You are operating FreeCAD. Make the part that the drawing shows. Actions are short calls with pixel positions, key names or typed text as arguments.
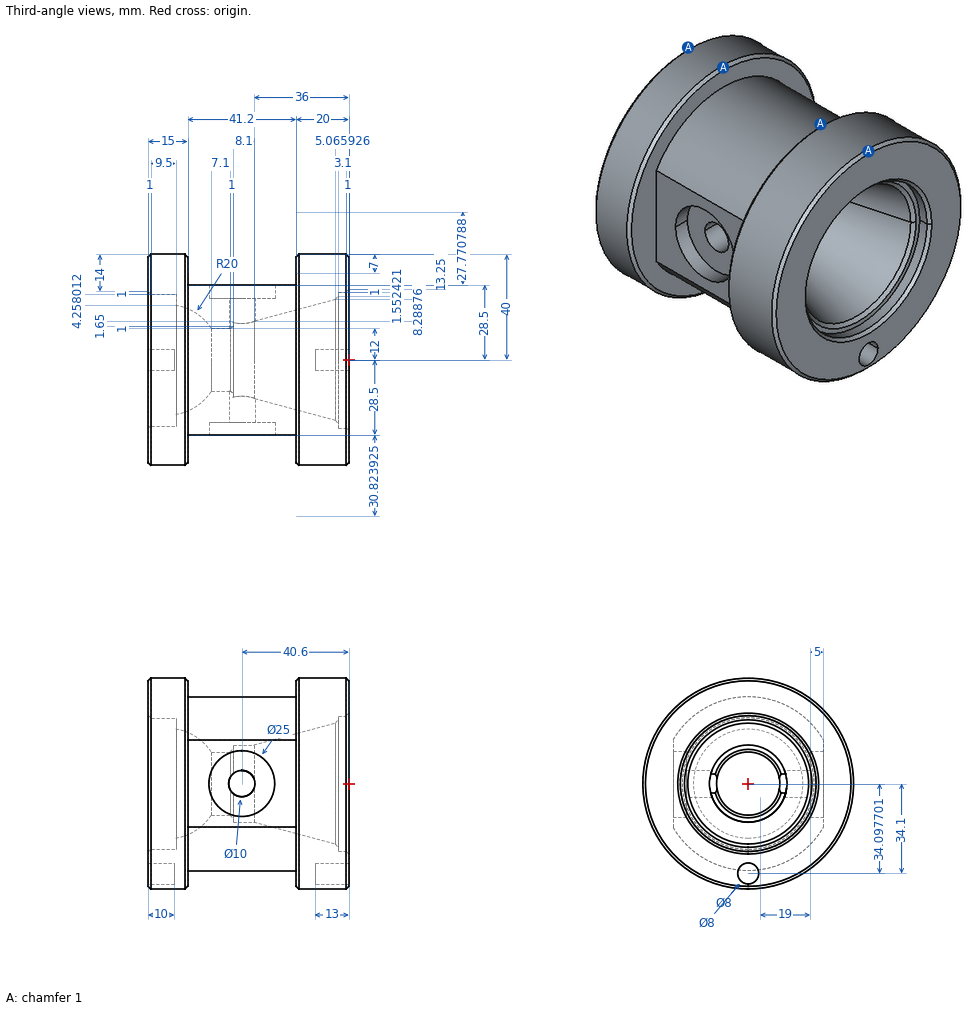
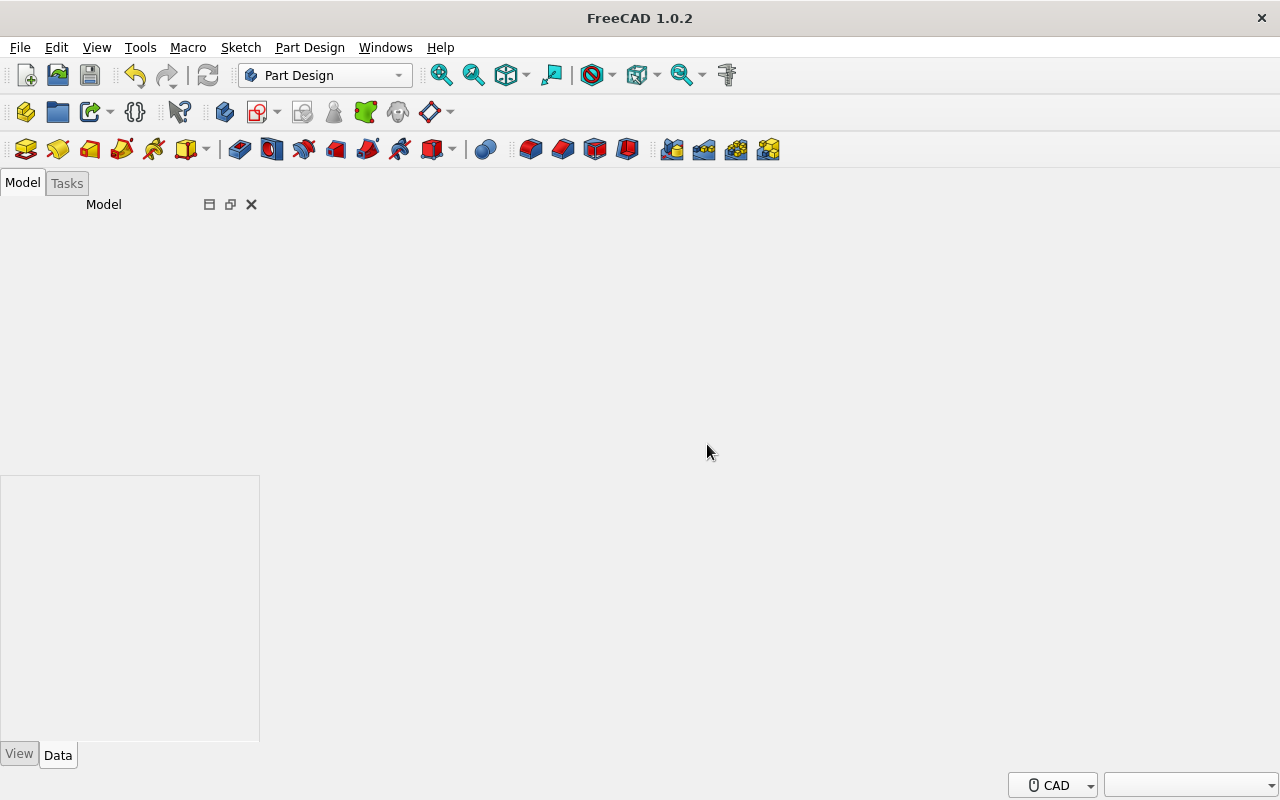
click(26, 76)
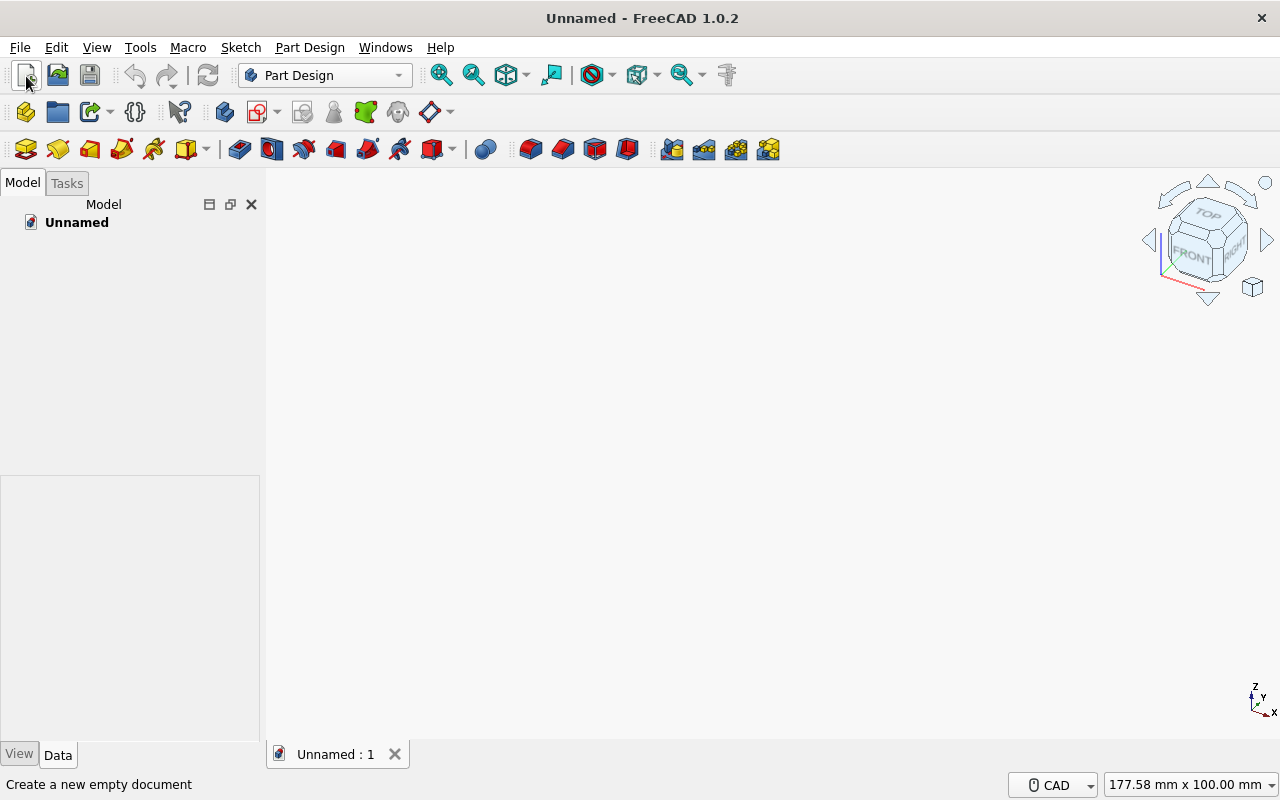
click(258, 112)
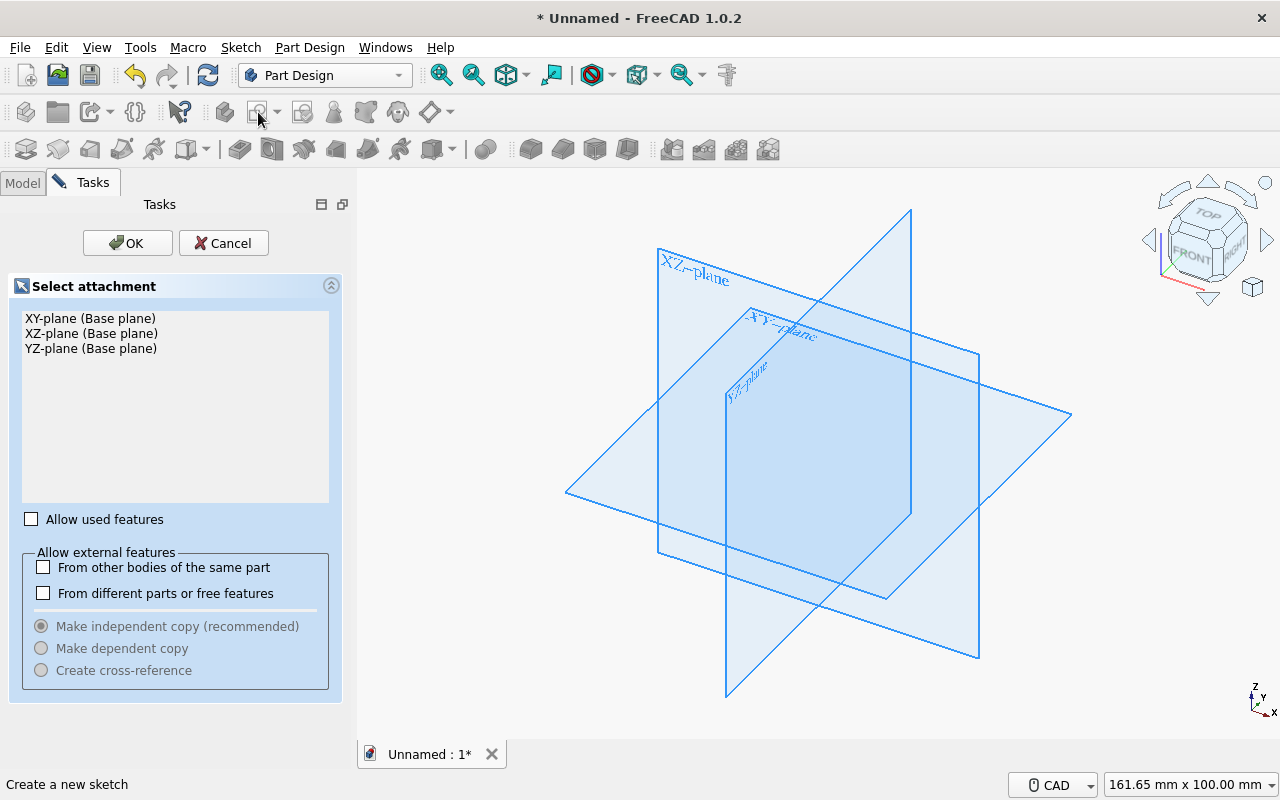
click(82, 318)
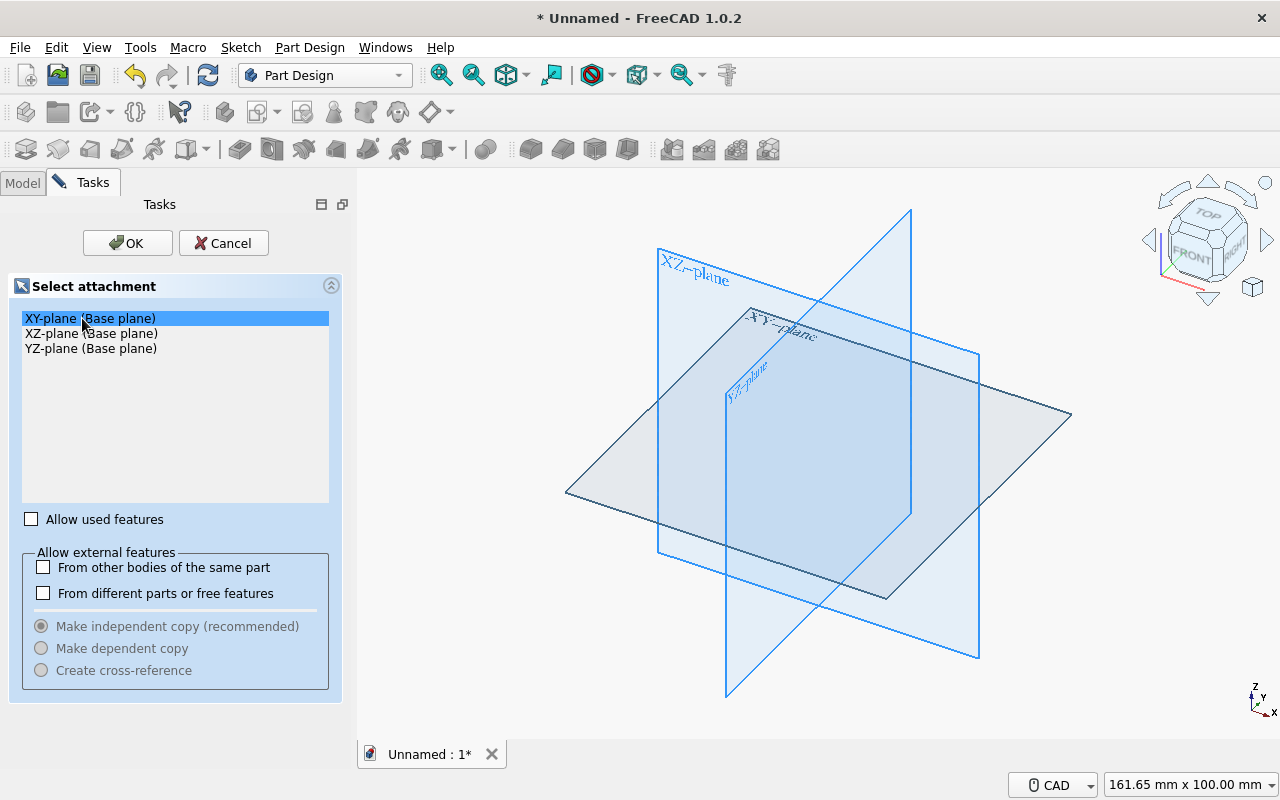
click(128, 243)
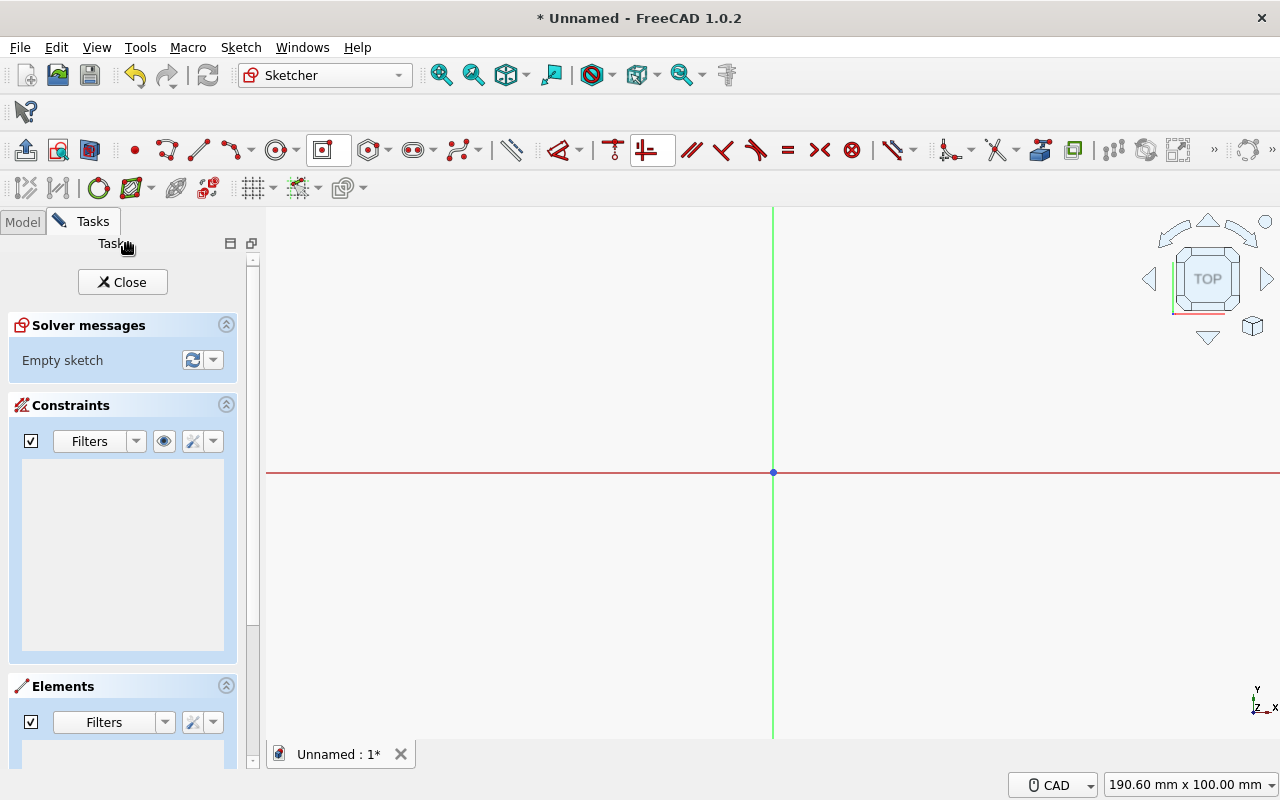
scroll(297, 235, up, 2)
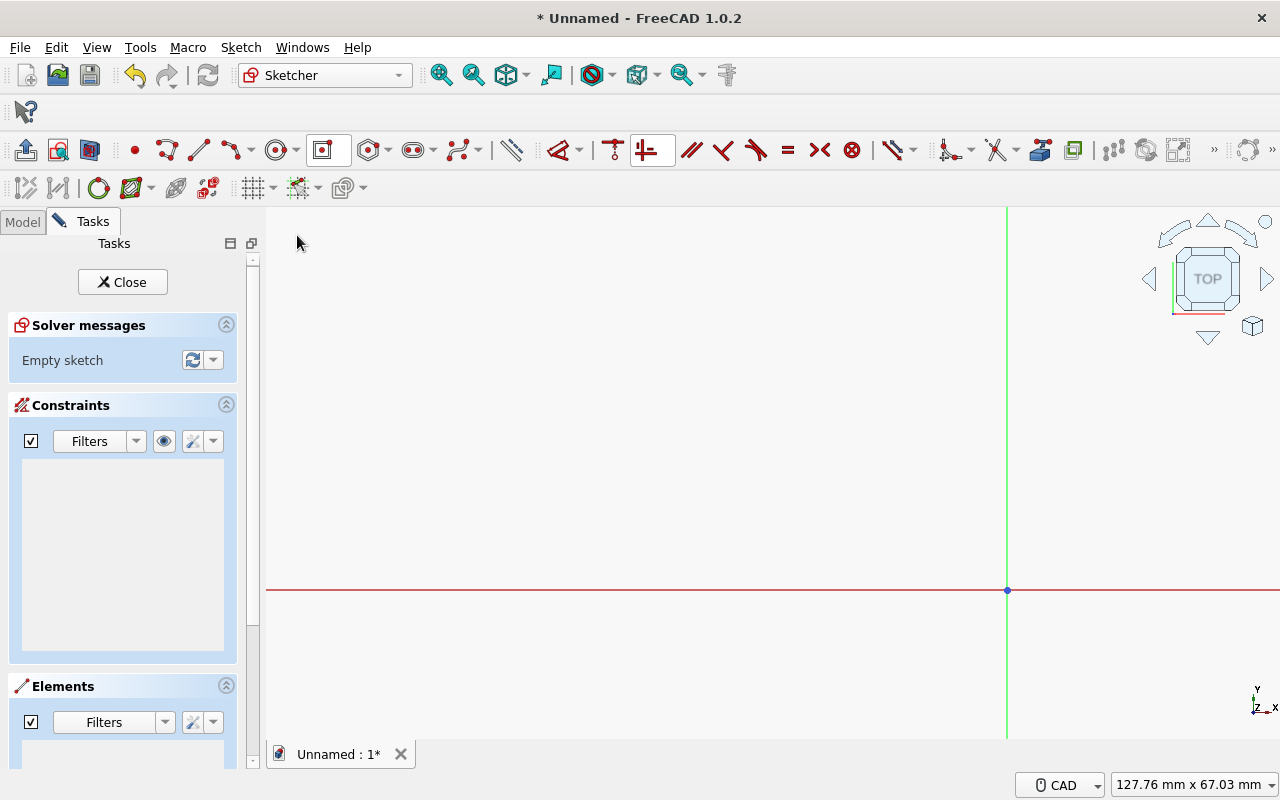
click(168, 150)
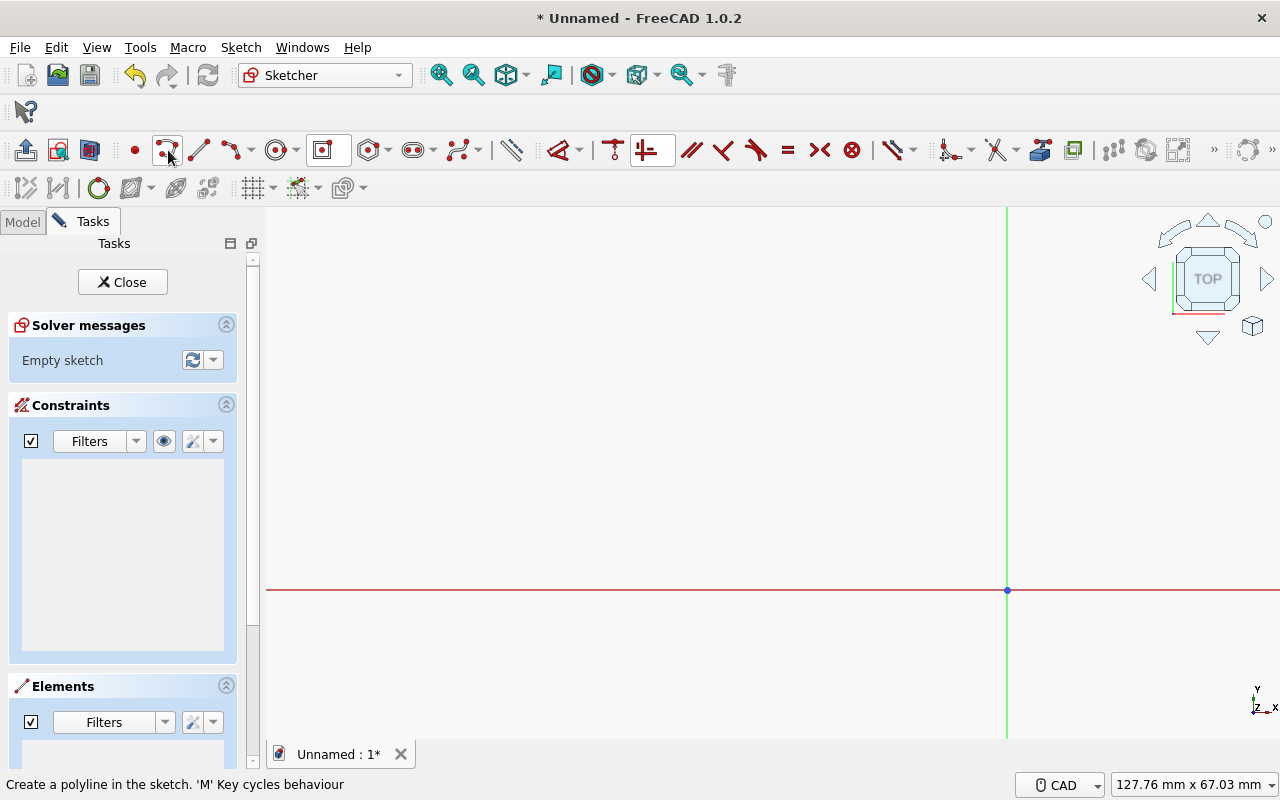
click(593, 495)
click(649, 495)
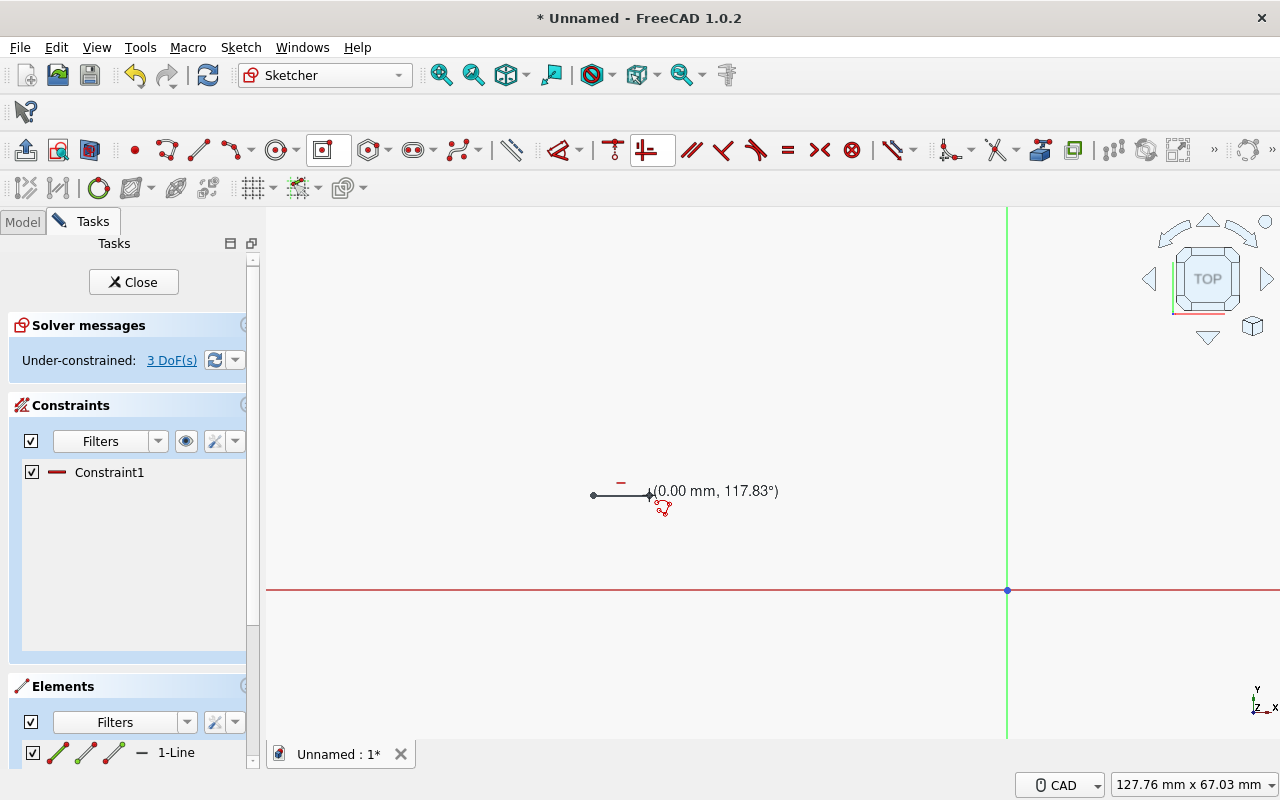
scroll(657, 487, up, 2)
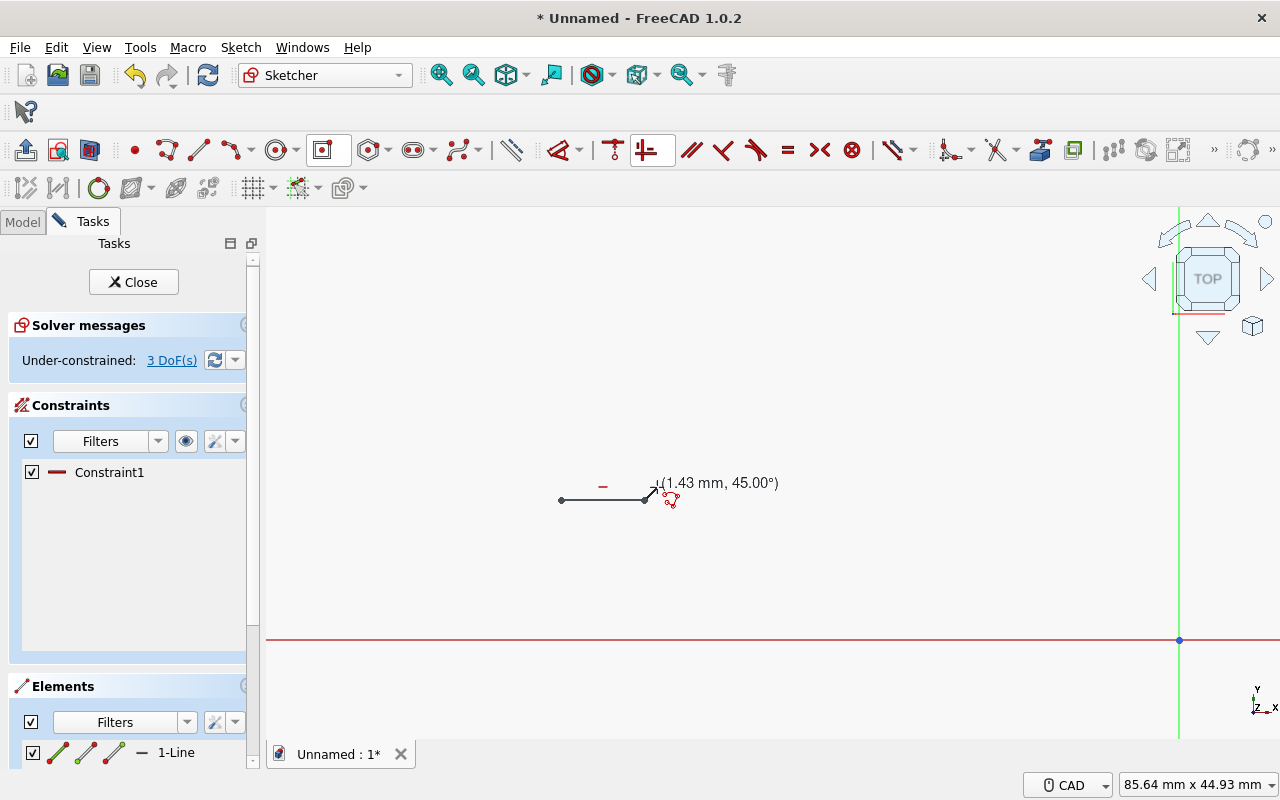
click(657, 487)
click(657, 467)
click(753, 467)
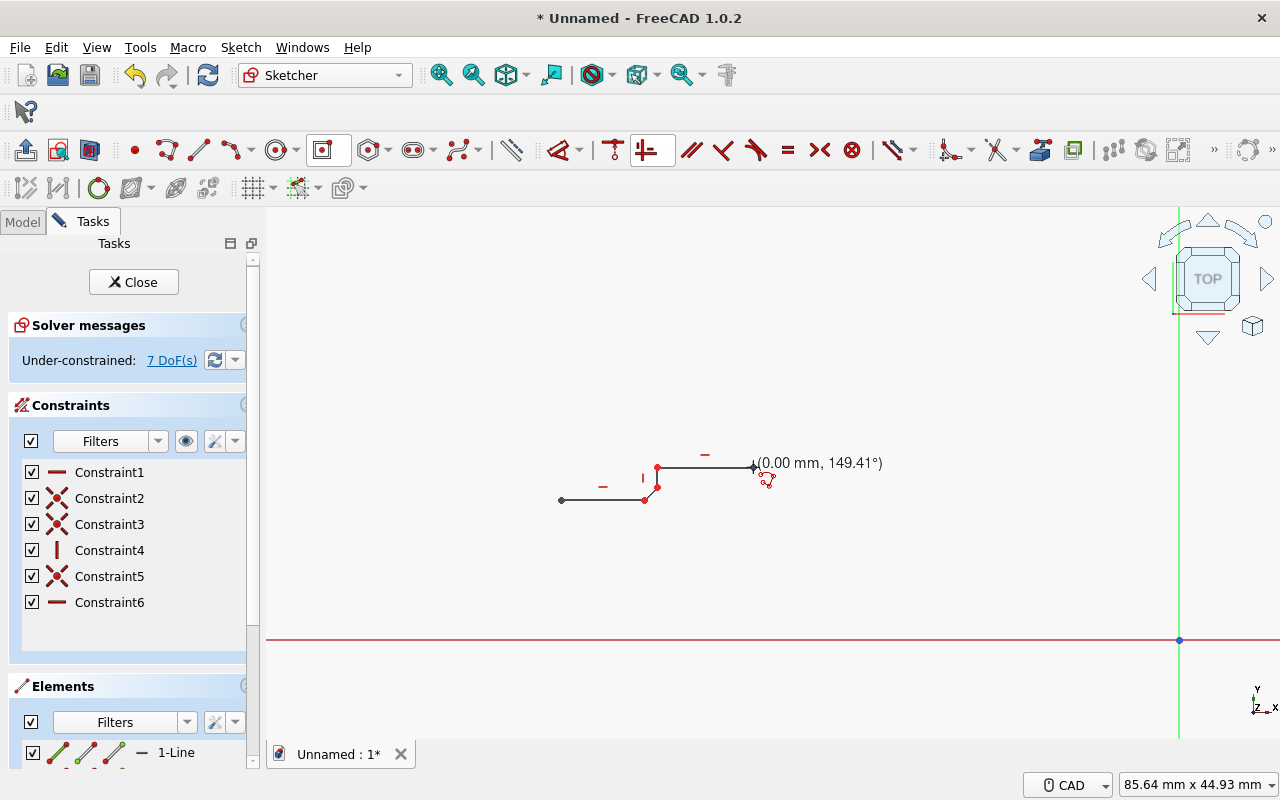
scroll(657, 614, down, 2)